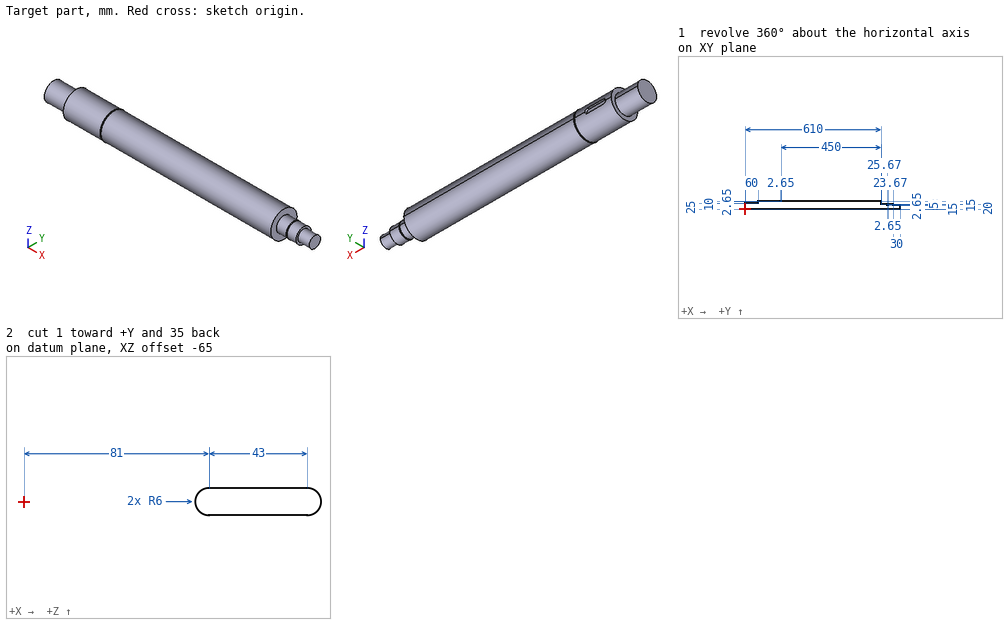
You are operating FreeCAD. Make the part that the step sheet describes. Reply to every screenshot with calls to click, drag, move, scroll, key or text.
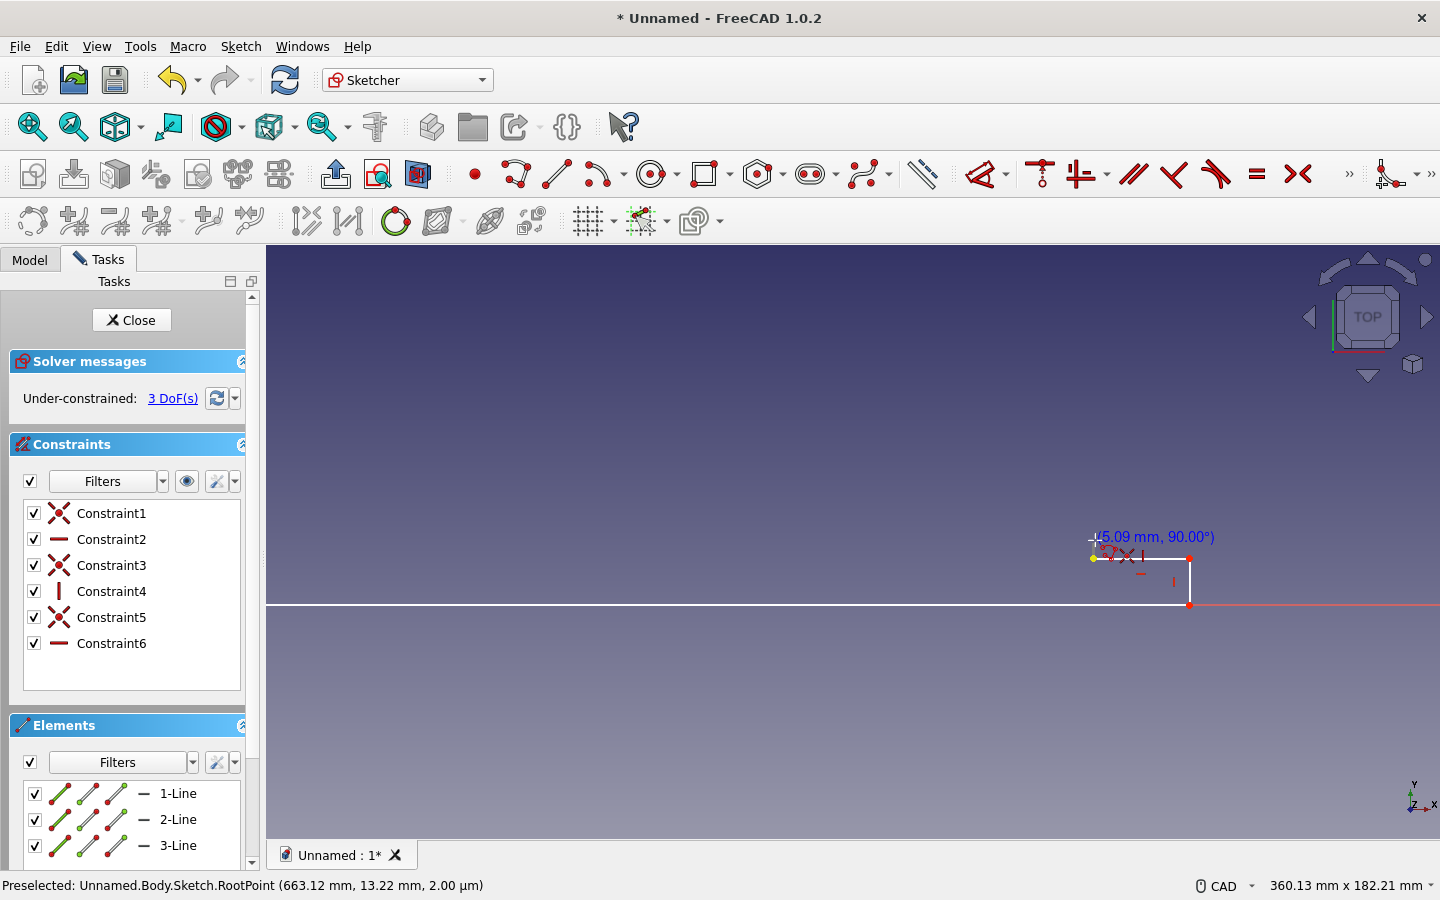
click(1093, 540)
click(1016, 540)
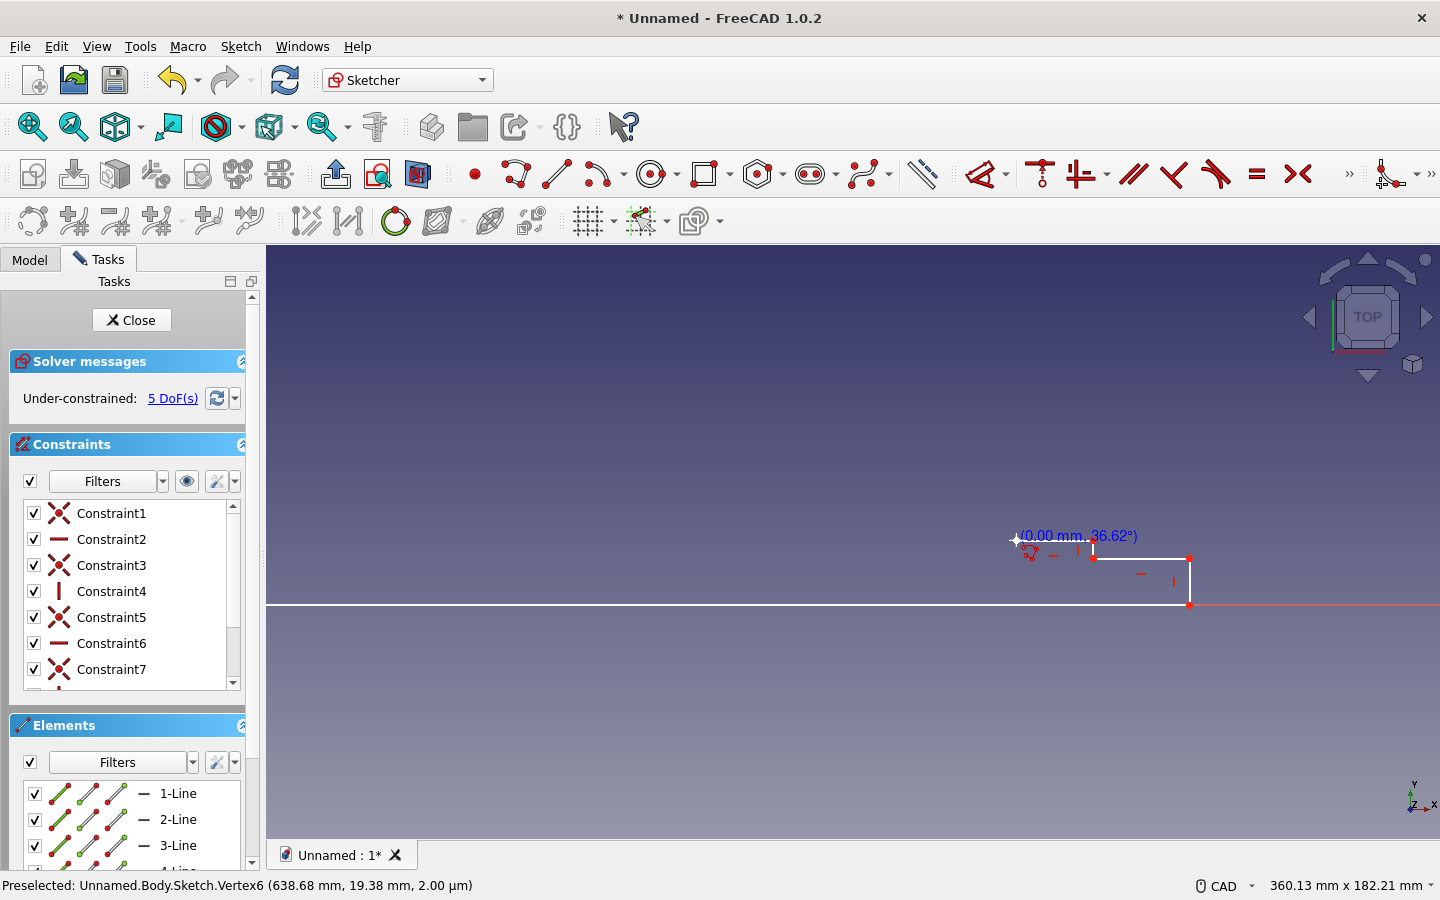
scroll(1016, 549, up, 4)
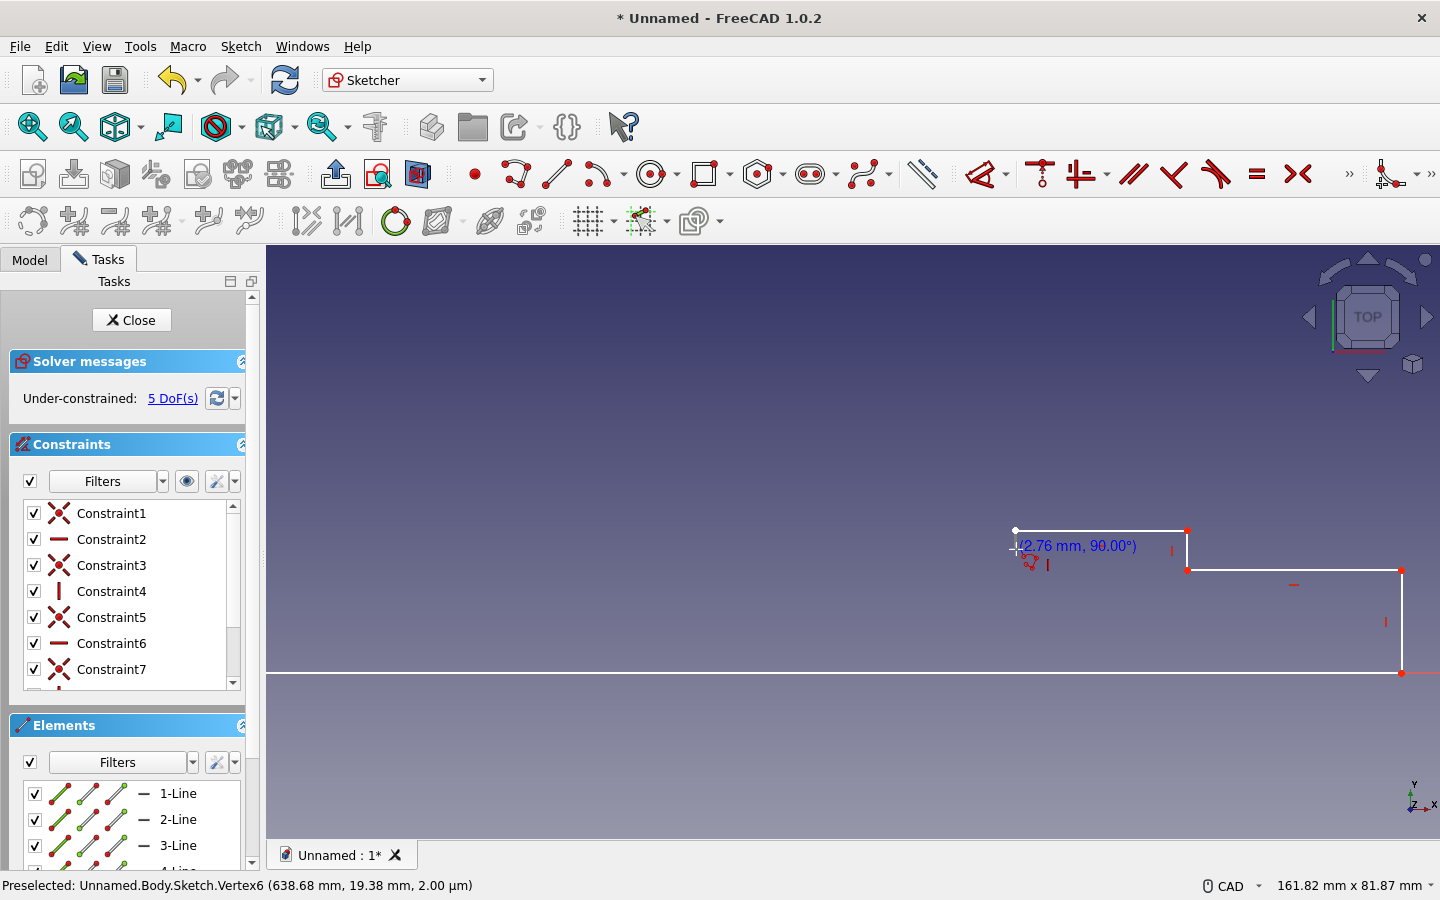
click(1015, 548)
click(996, 548)
click(996, 528)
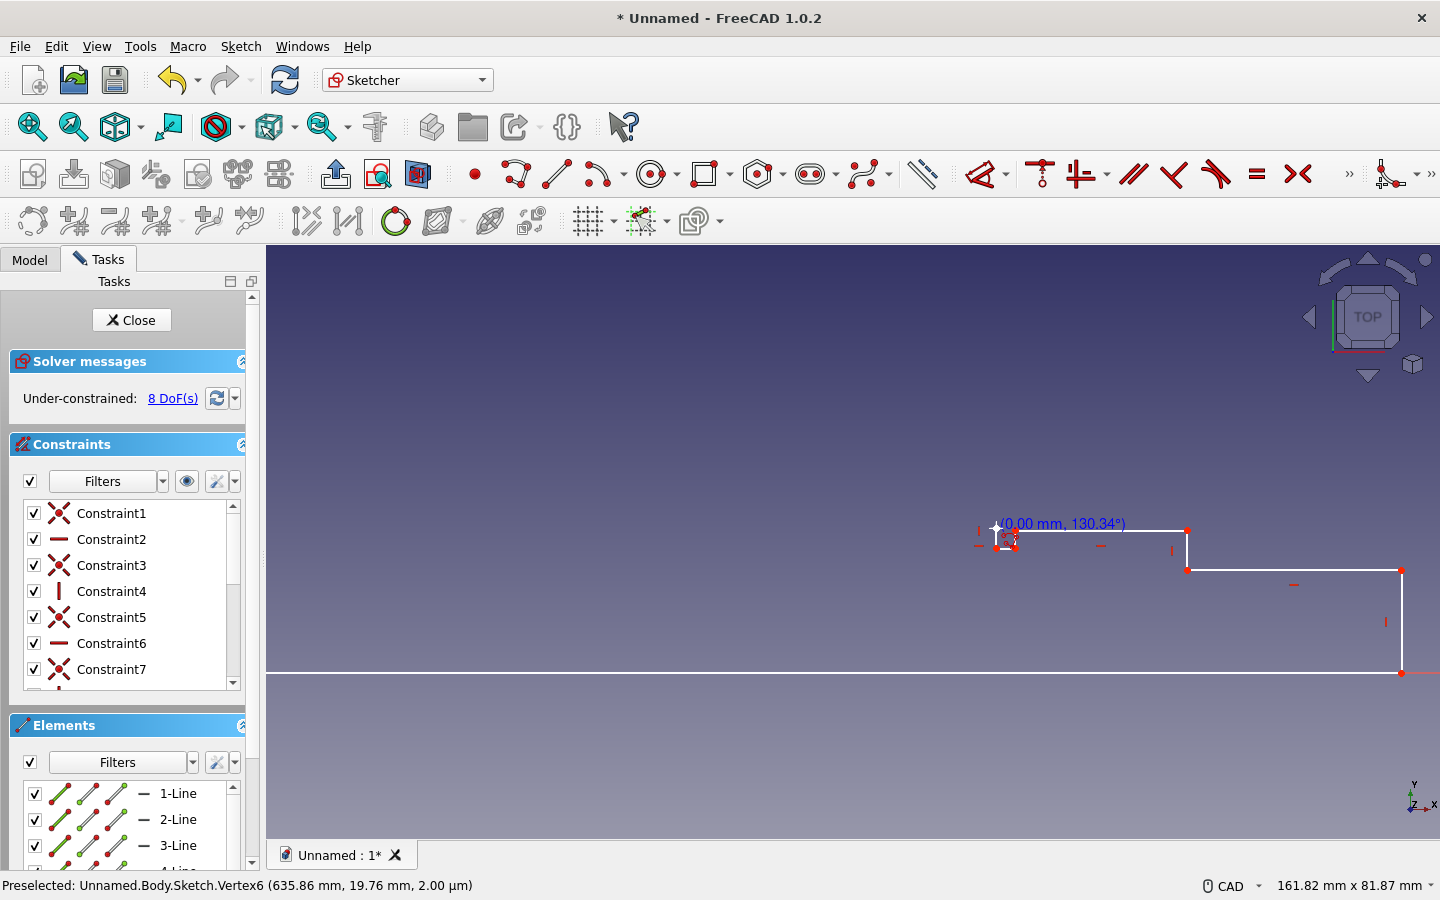
scroll(1080, 541, down, 10)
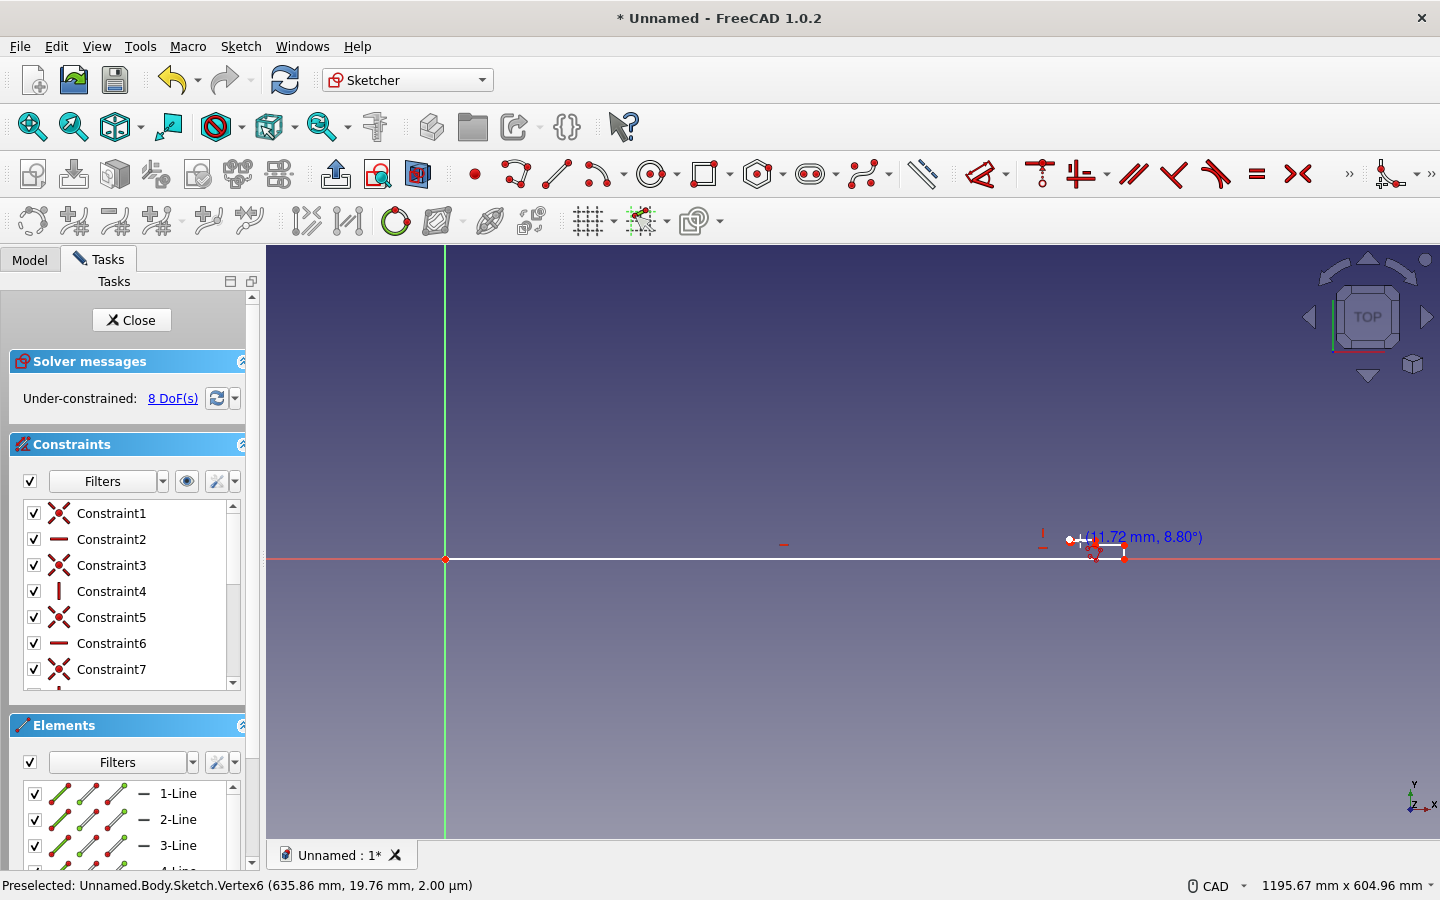
click(1044, 540)
click(1044, 525)
click(602, 525)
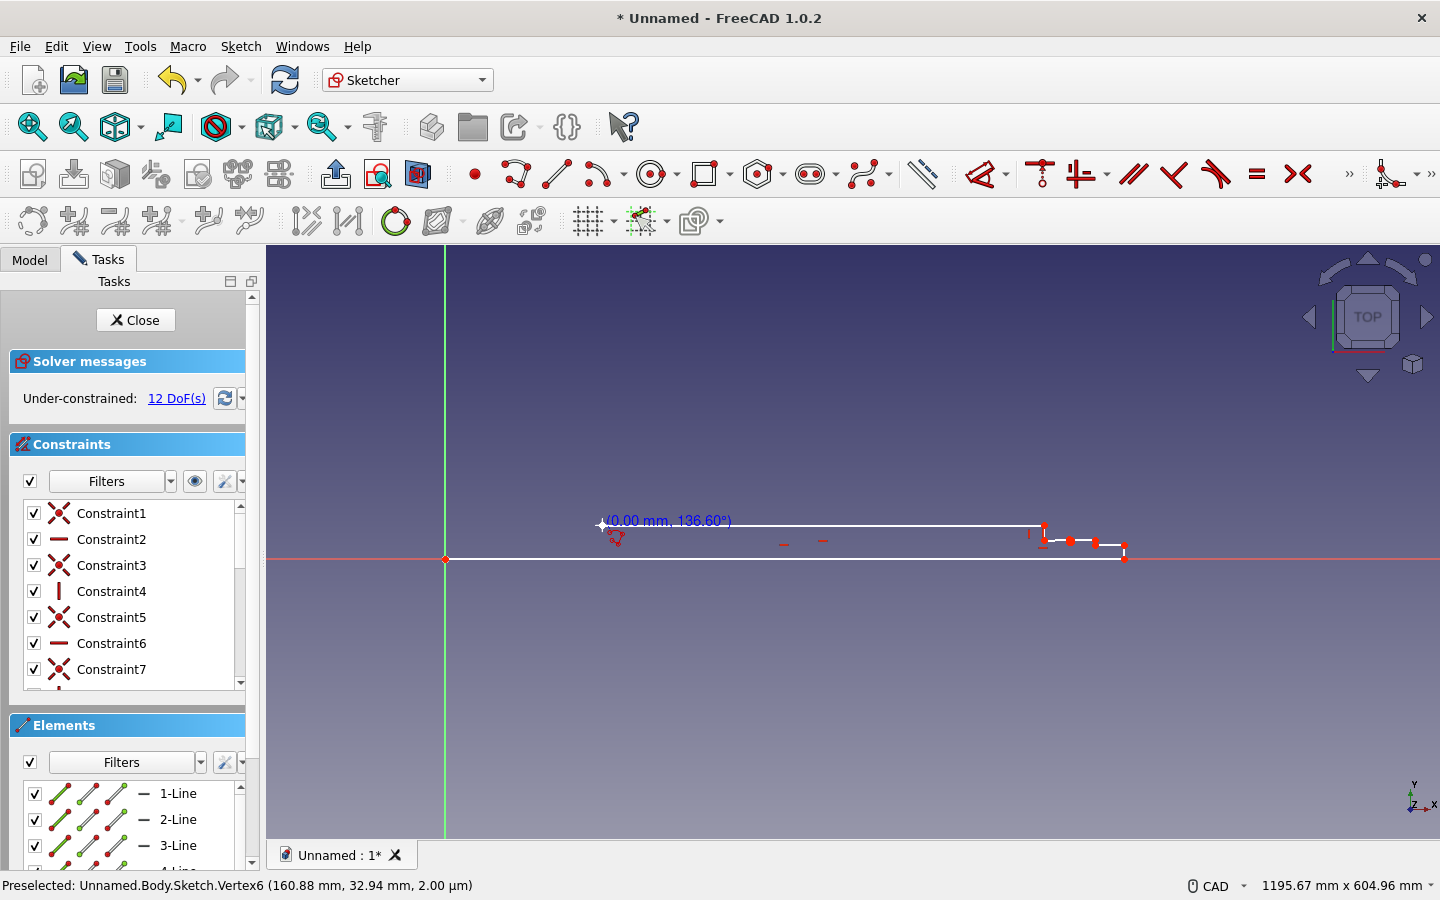
scroll(602, 528, up, 10)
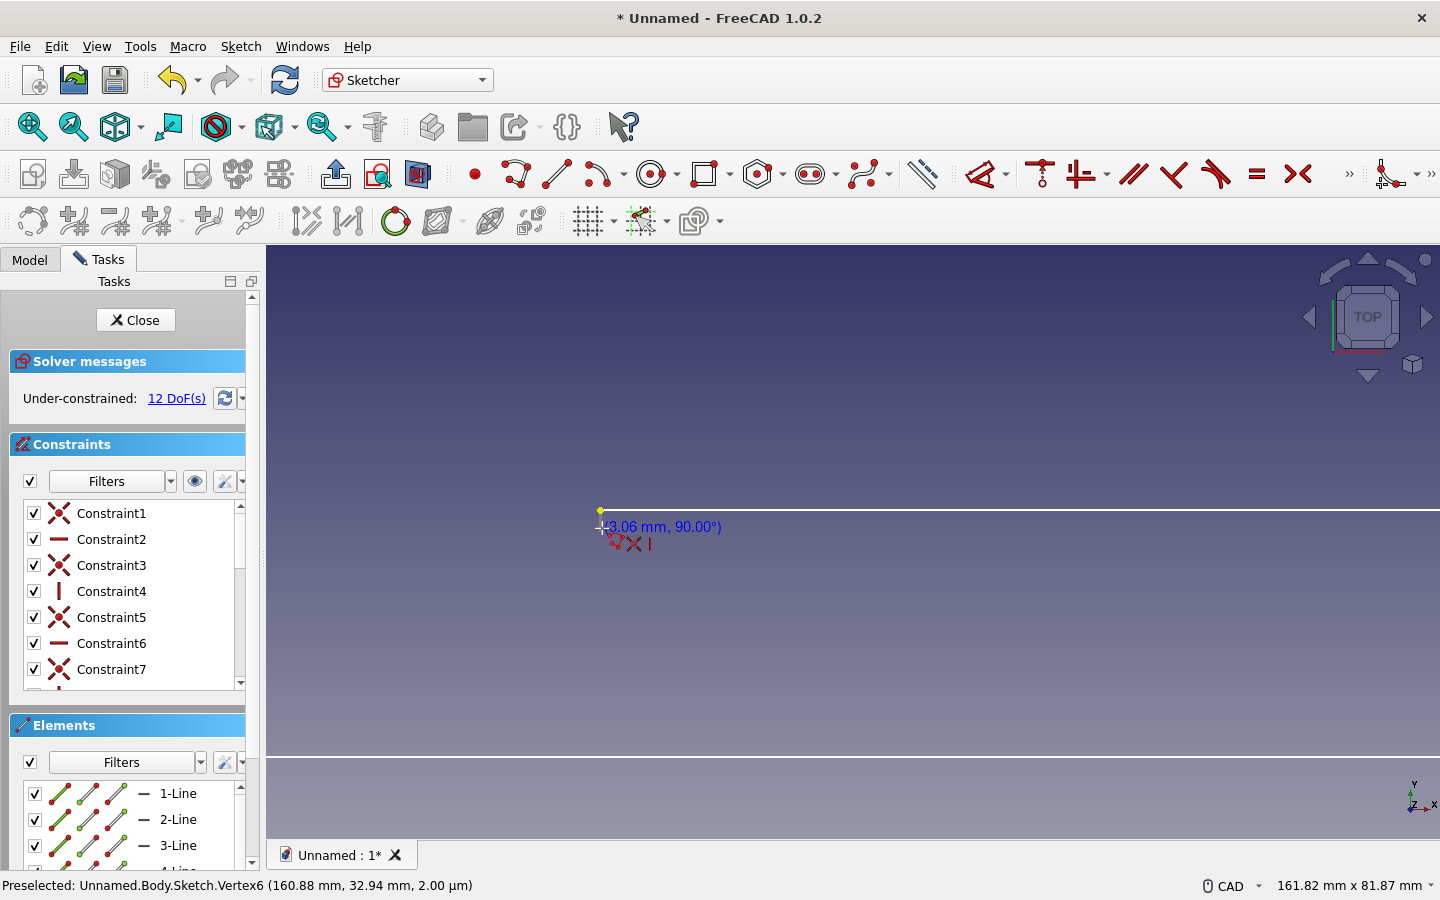
click(600, 522)
click(582, 522)
click(582, 503)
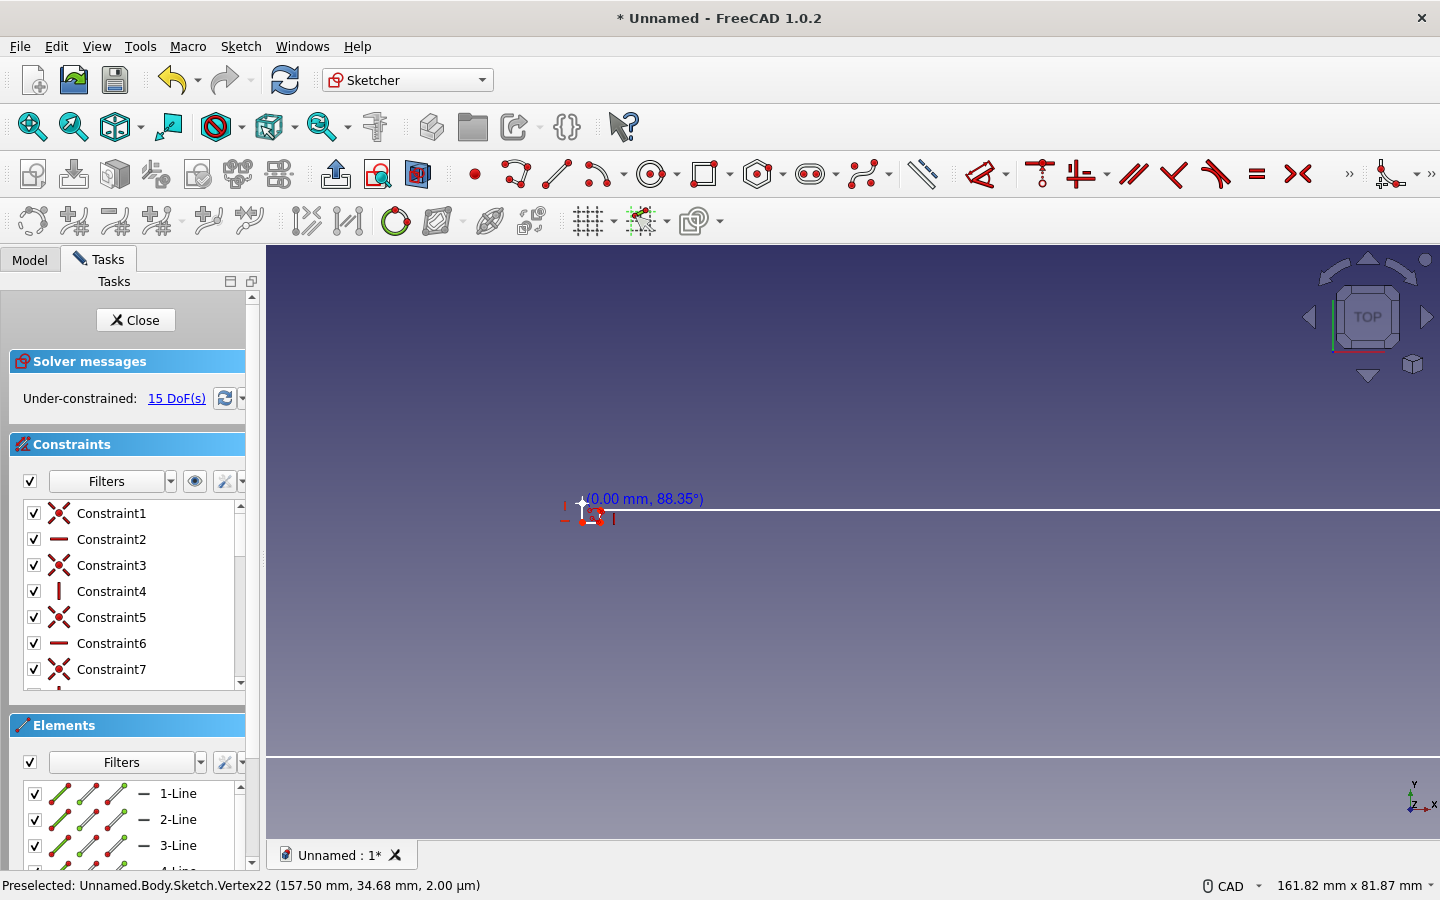
scroll(602, 528, down, 10)